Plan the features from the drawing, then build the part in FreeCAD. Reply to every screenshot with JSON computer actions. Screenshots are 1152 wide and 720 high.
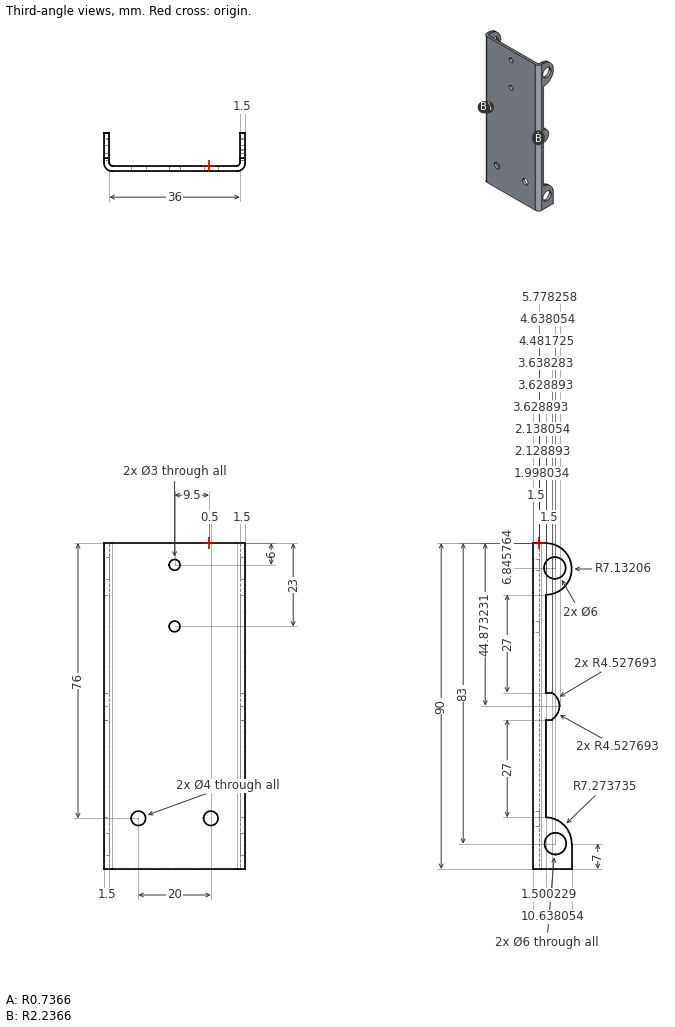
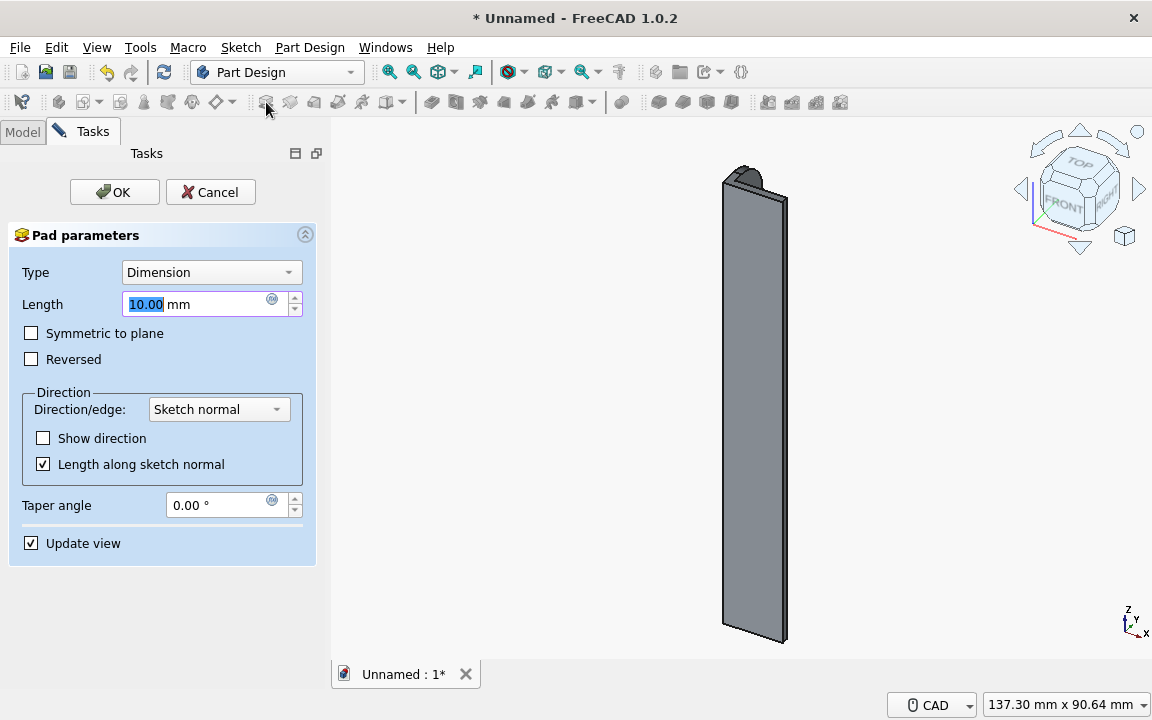
{"action": "type", "text": "36"}
{"action": "key", "text": "Tab"}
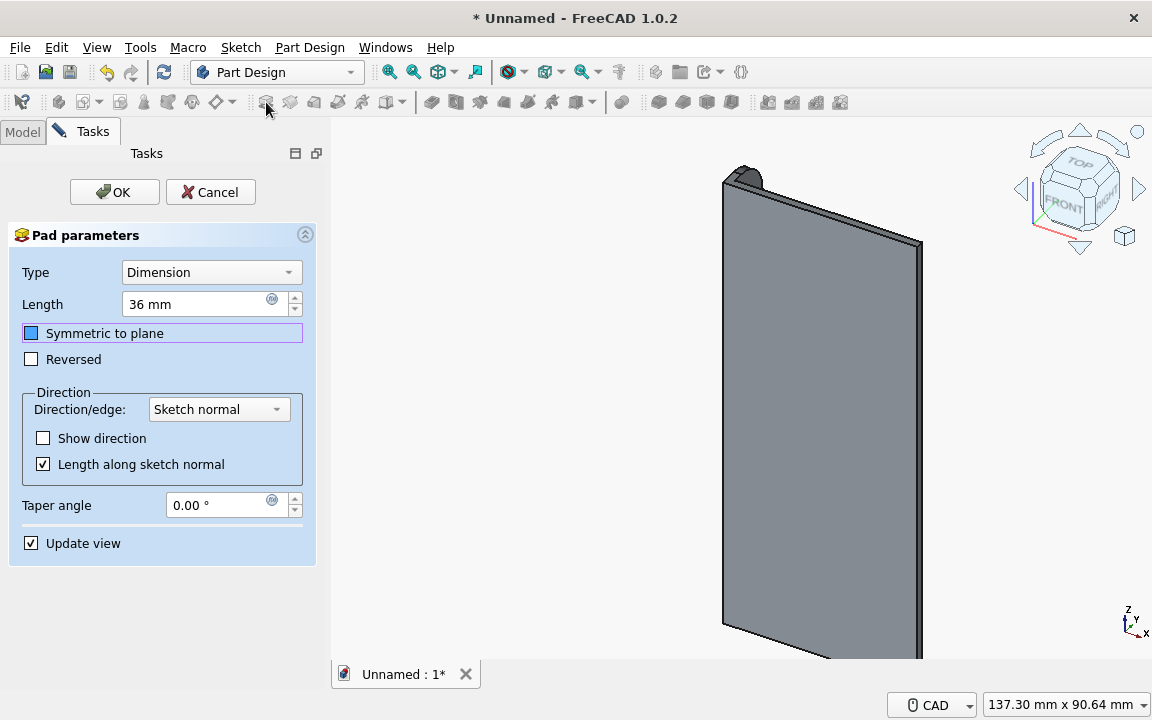
{"action": "left_click", "coordinate": [115, 192]}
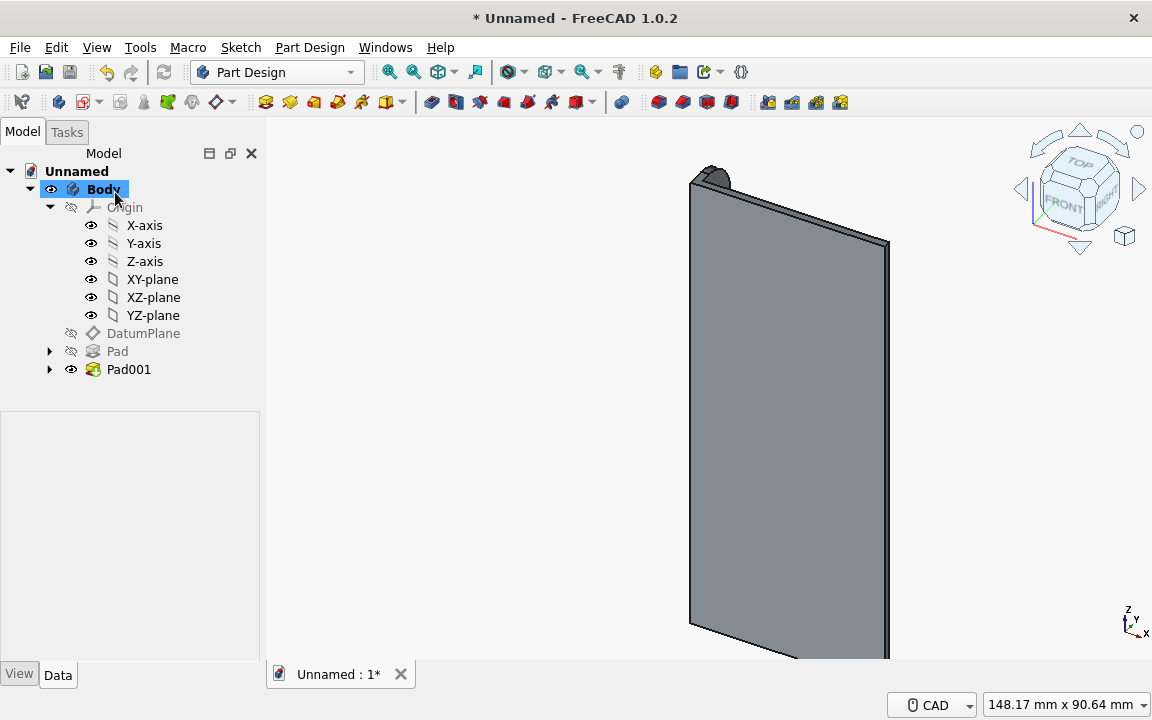
{"action": "key", "text": "v f"}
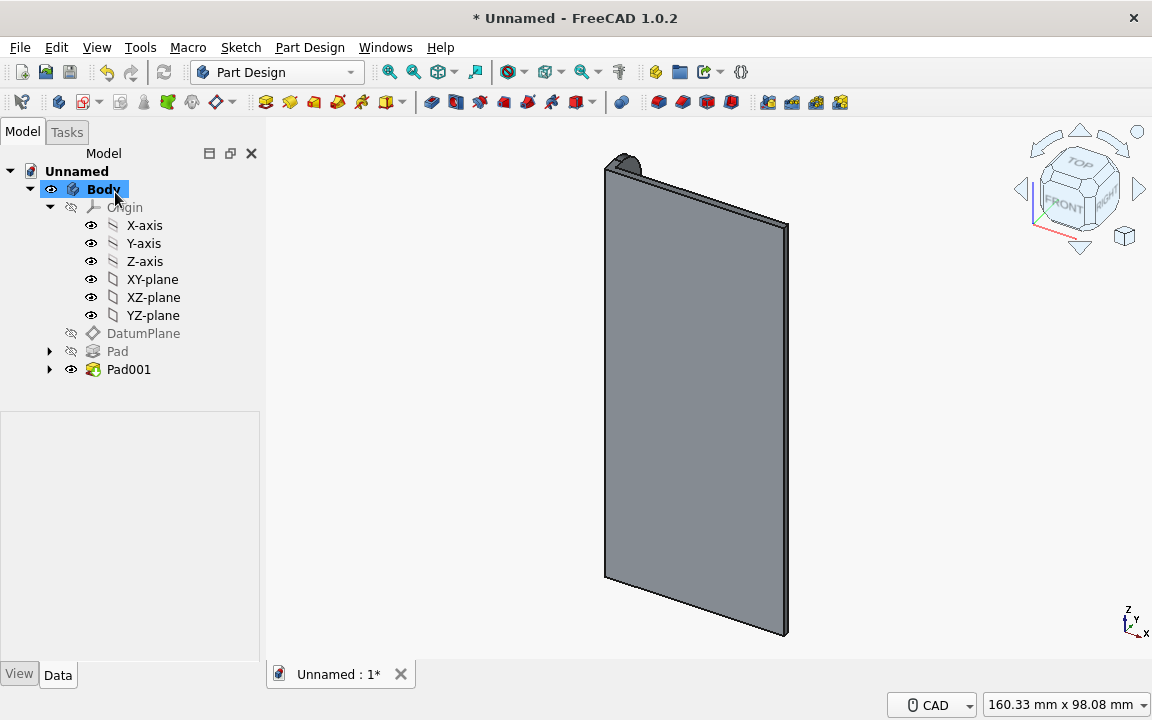
{"action": "scroll", "coordinate": [786, 255], "scroll_direction": "up", "scroll_amount": 6}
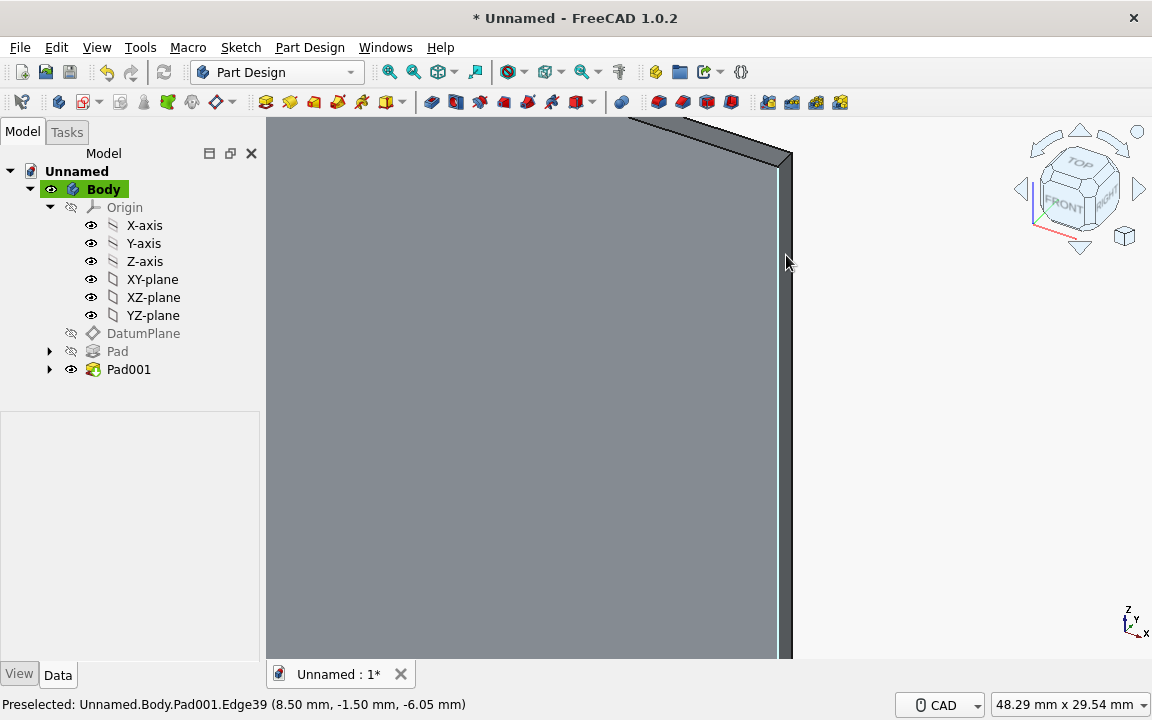
{"action": "key", "text": "v f"}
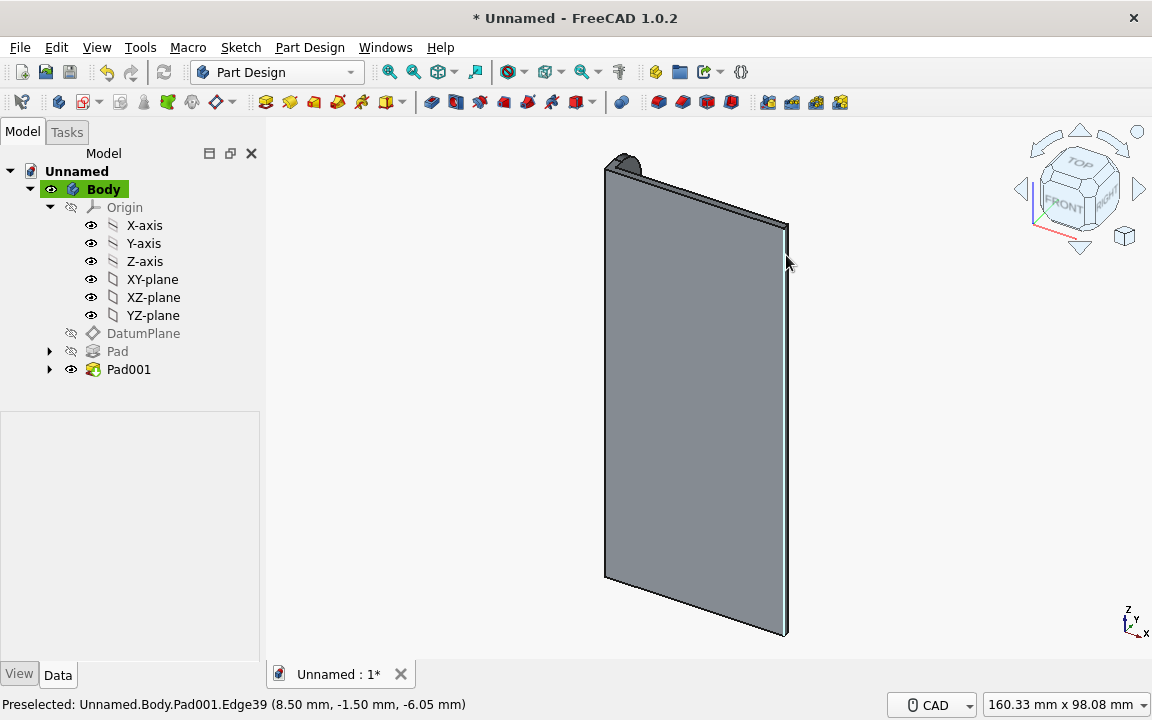
{"action": "key", "text": "0"}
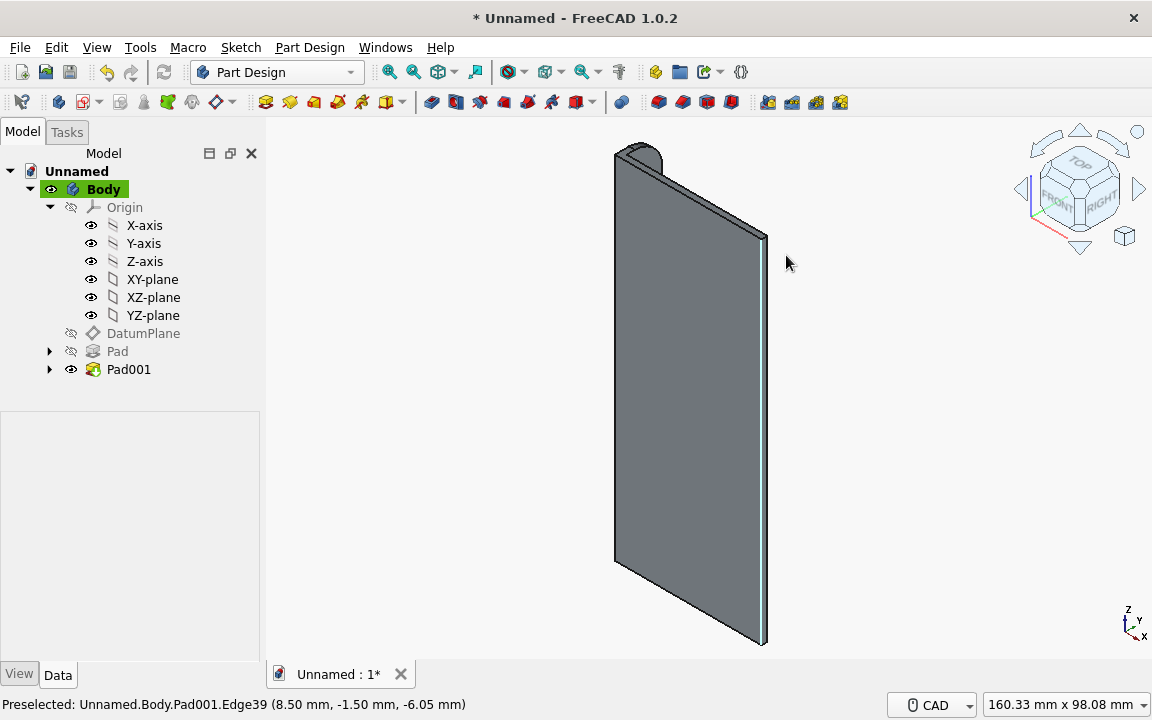
{"action": "scroll", "coordinate": [764, 266], "scroll_direction": "up", "scroll_amount": 6}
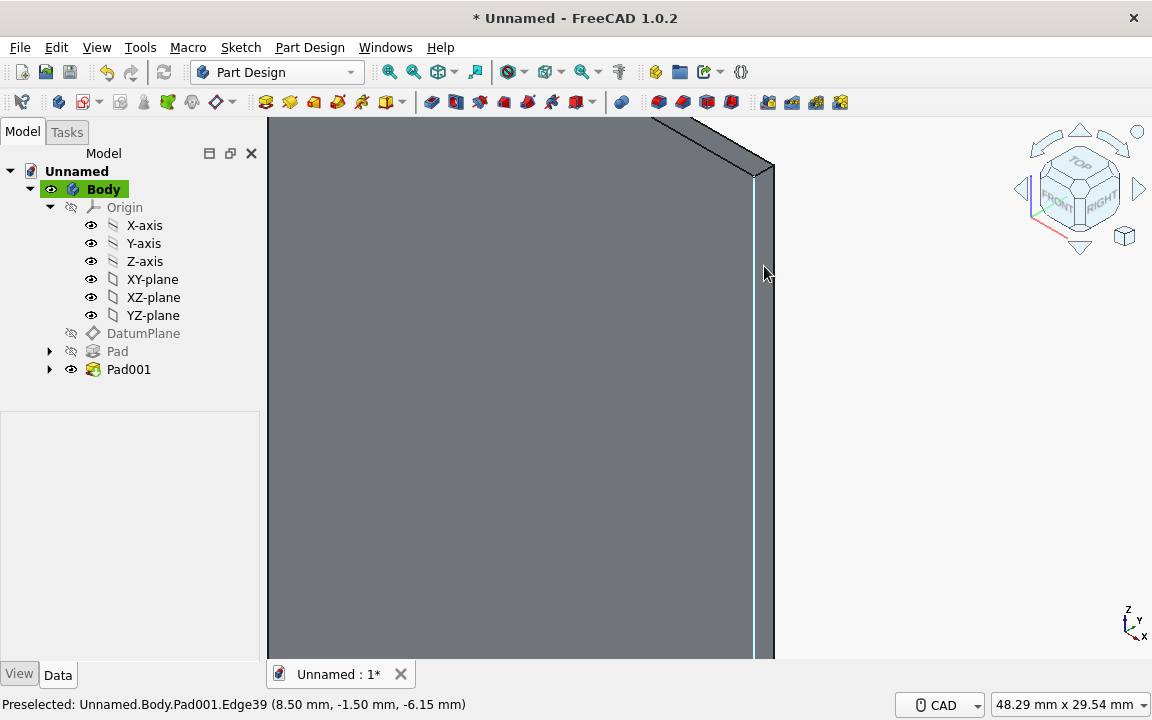
{"action": "left_click", "coordinate": [764, 266]}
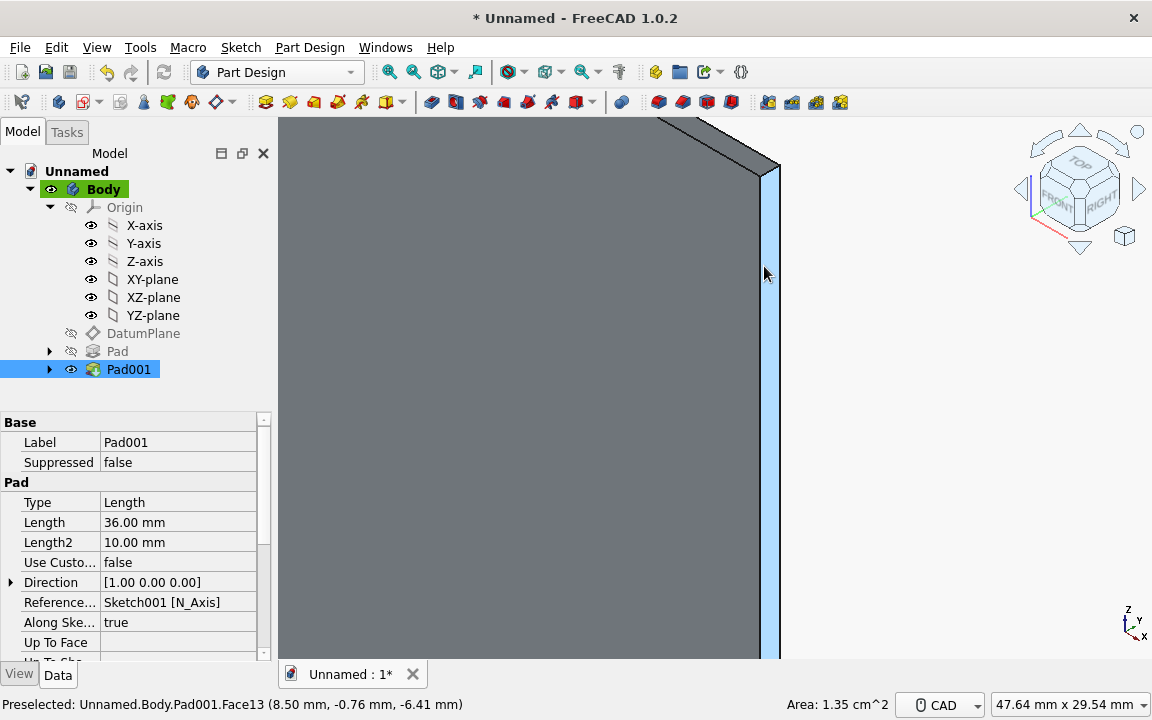
{"action": "left_click", "coordinate": [84, 102]}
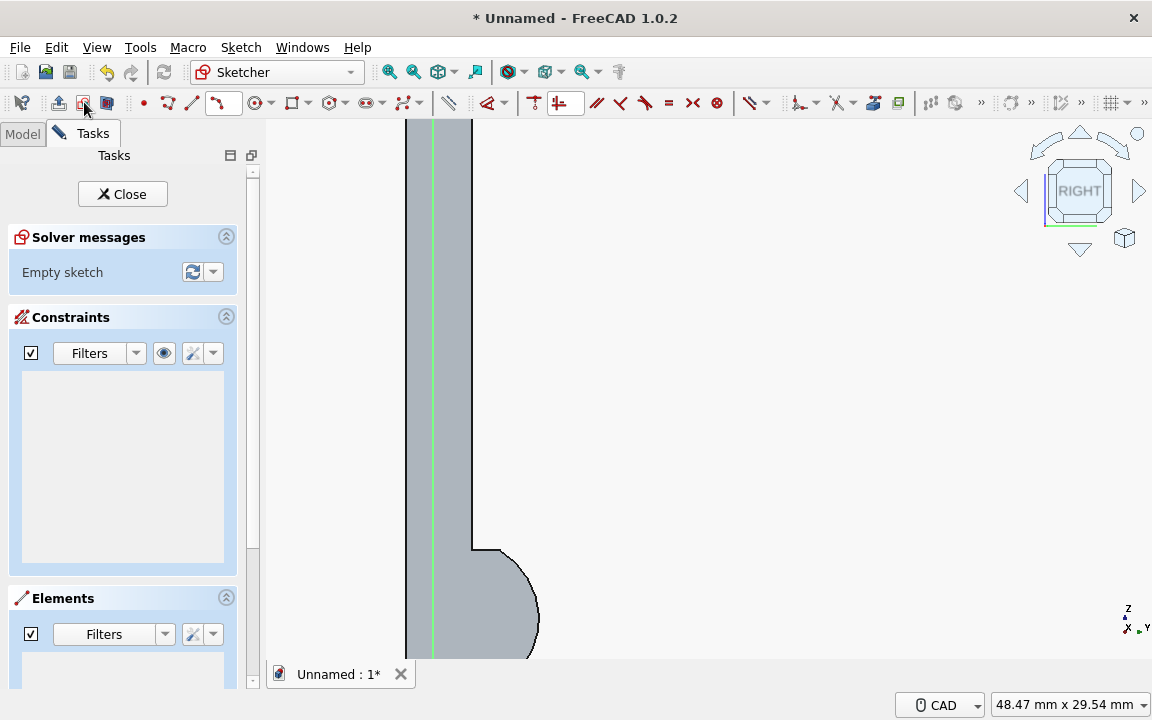
{"action": "scroll", "coordinate": [675, 331], "scroll_direction": "down", "scroll_amount": 8}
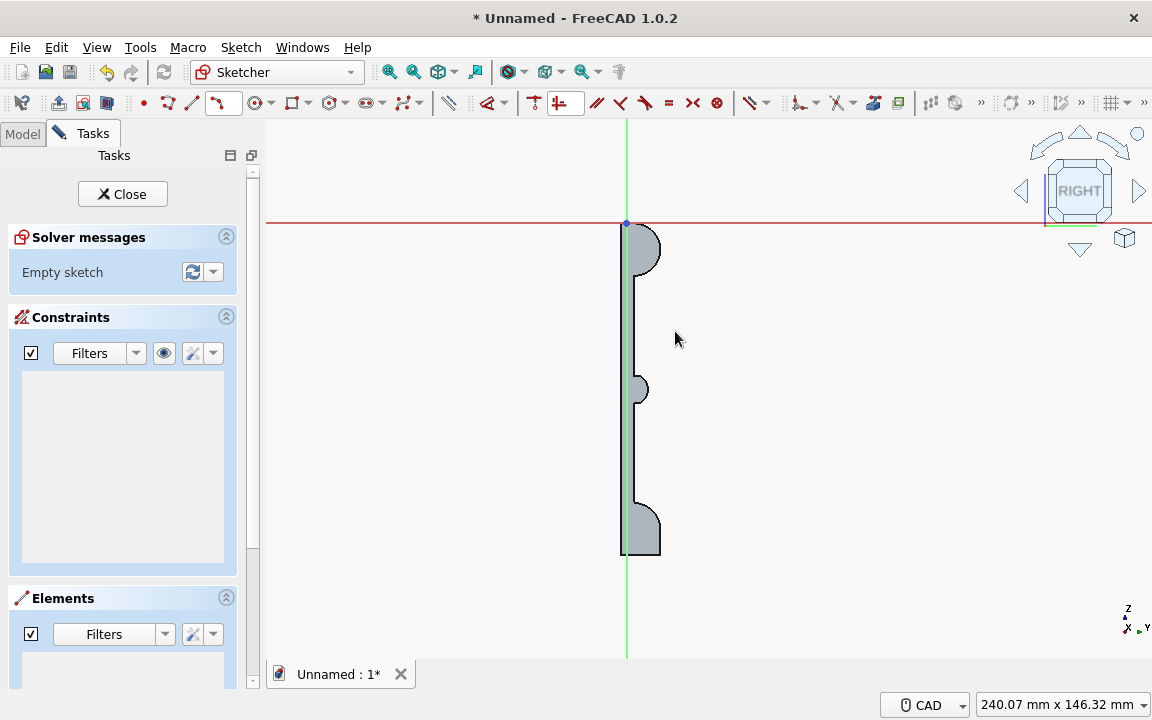
{"action": "key", "text": "g m"}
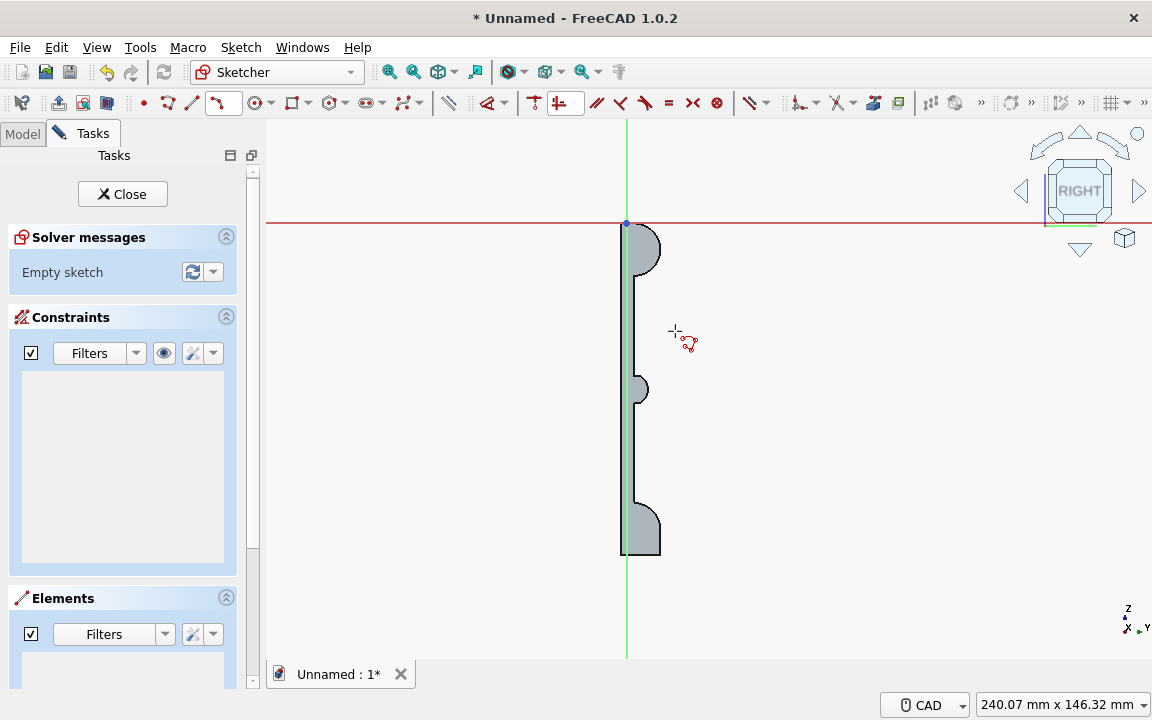
{"action": "scroll", "coordinate": [634, 223], "scroll_direction": "up", "scroll_amount": 4}